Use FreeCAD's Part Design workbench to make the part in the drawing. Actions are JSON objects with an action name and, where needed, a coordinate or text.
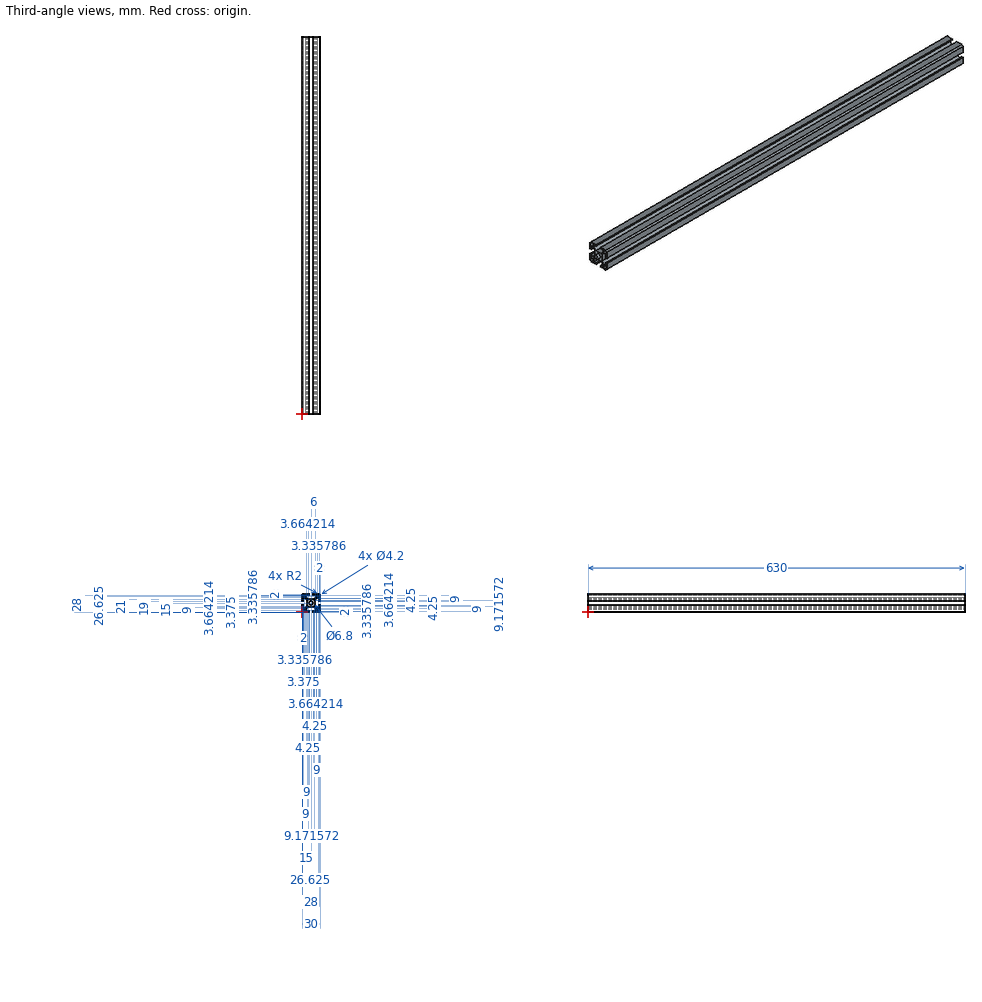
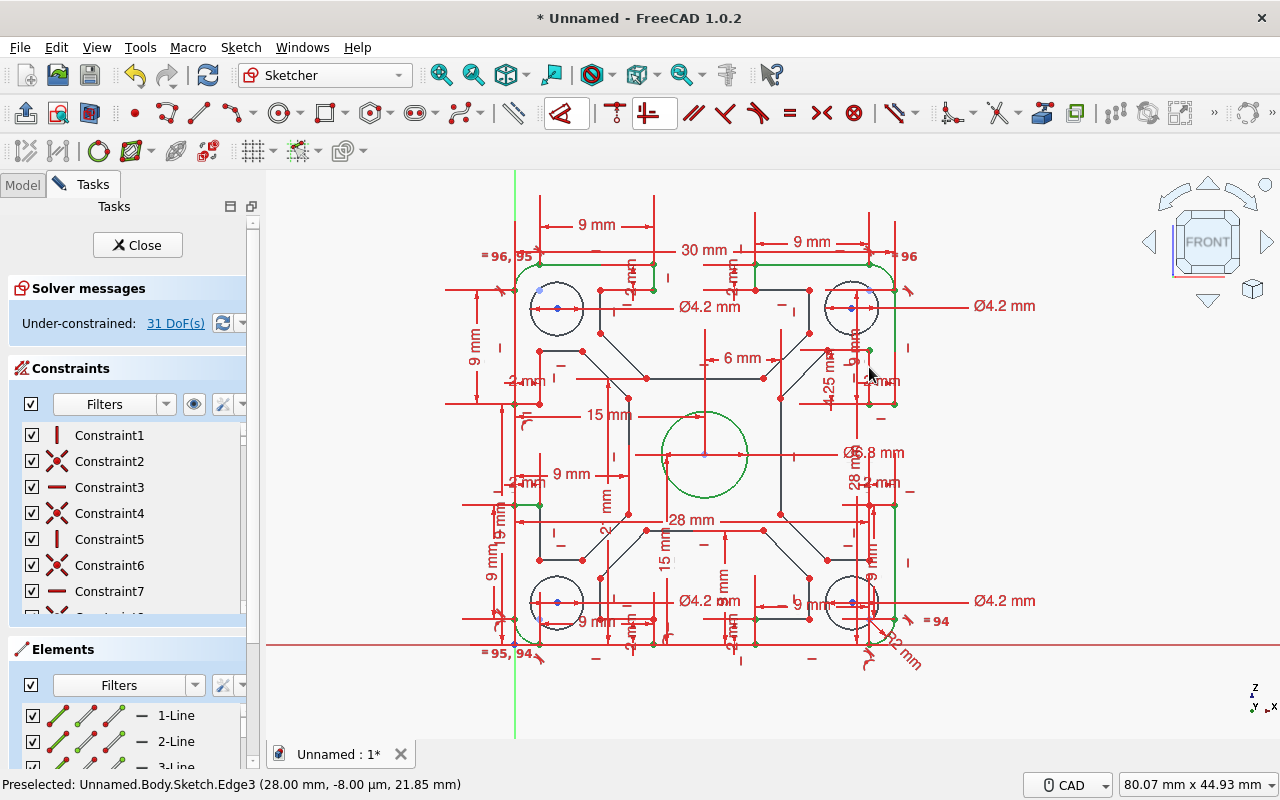
{"action": "left_click", "coordinate": [869, 522]}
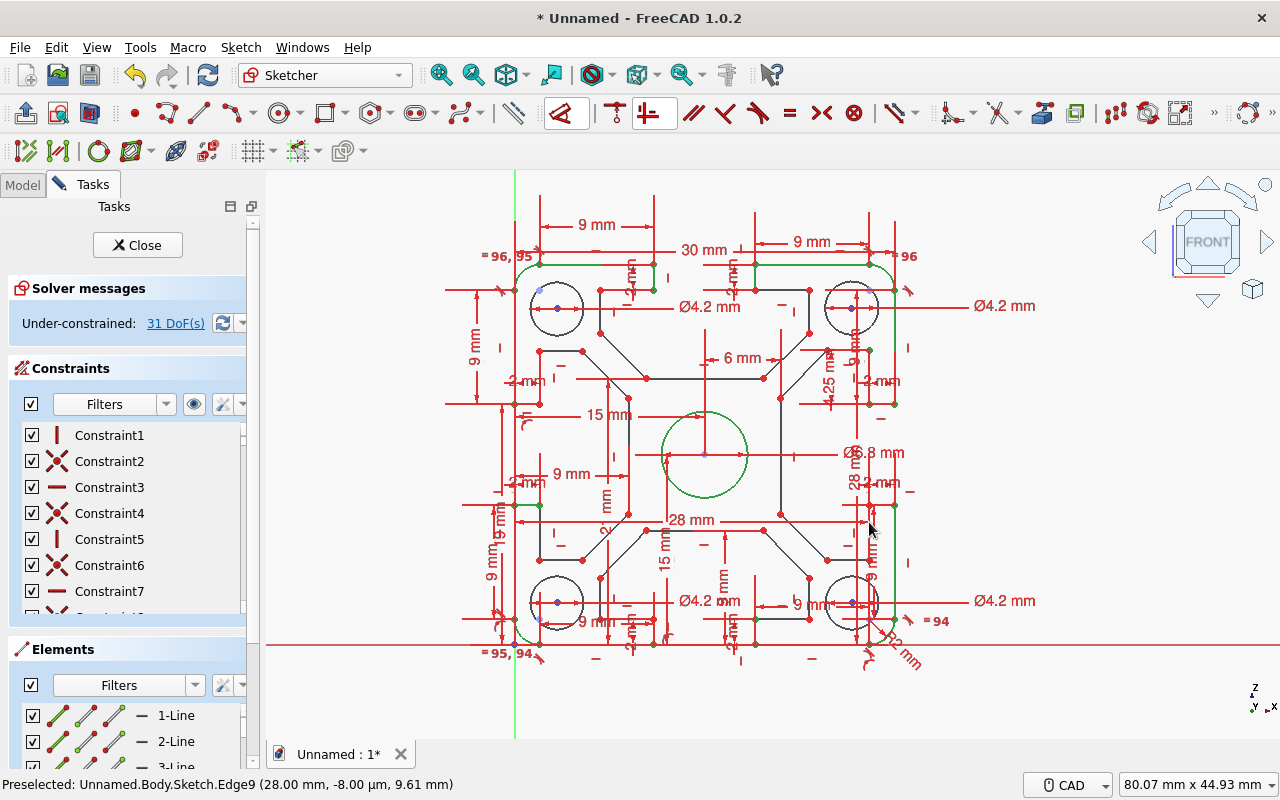
{"action": "key", "text": "i"}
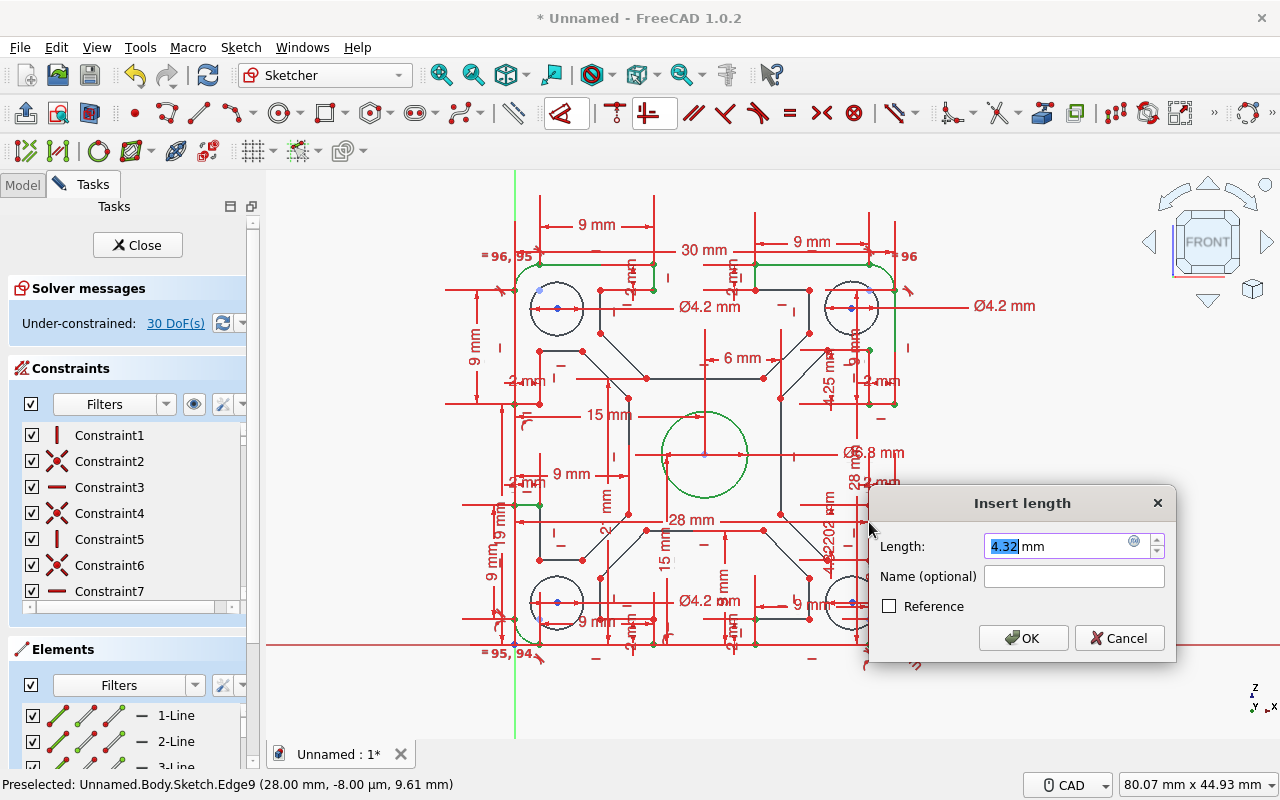
{"action": "type", "text": "4.25"}
{"action": "key", "text": "Return"}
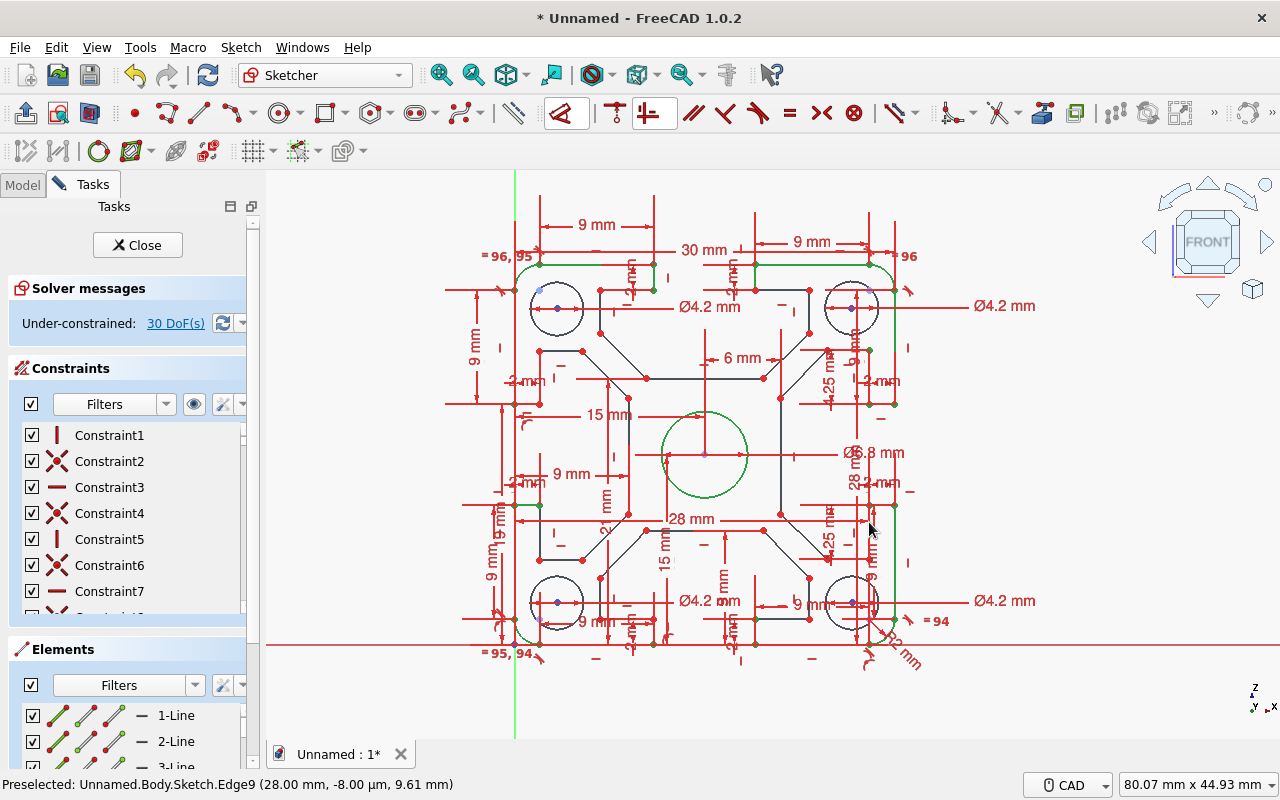
{"action": "left_click", "coordinate": [771, 619]}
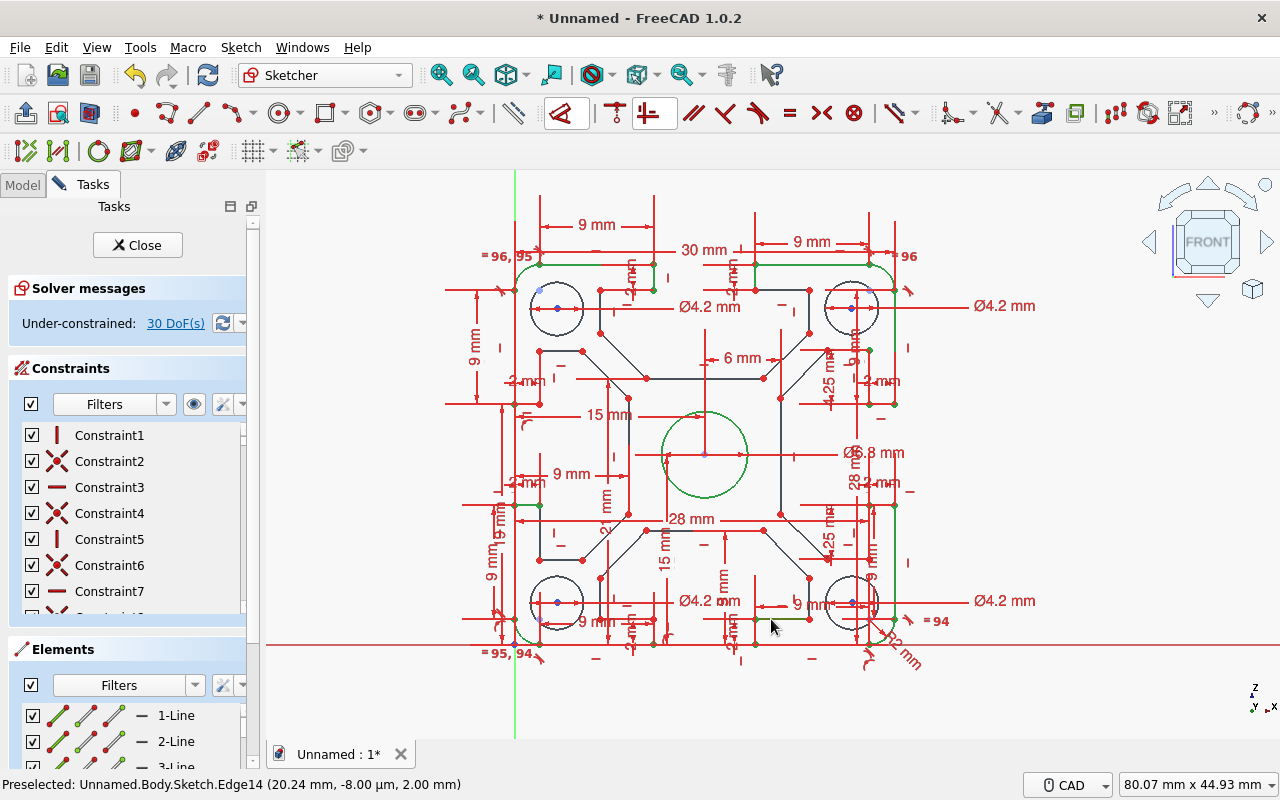
{"action": "key", "text": "l"}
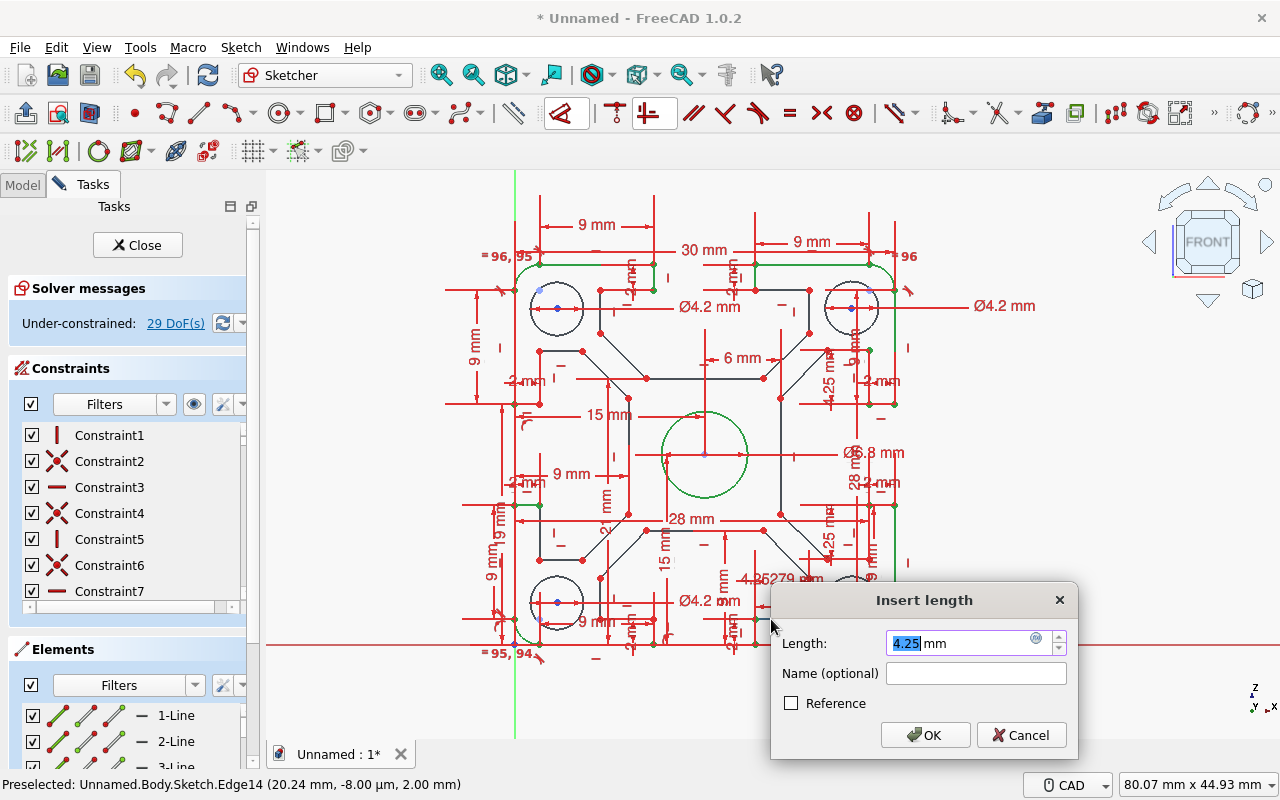
{"action": "type", "text": "4.25"}
{"action": "key", "text": "Return"}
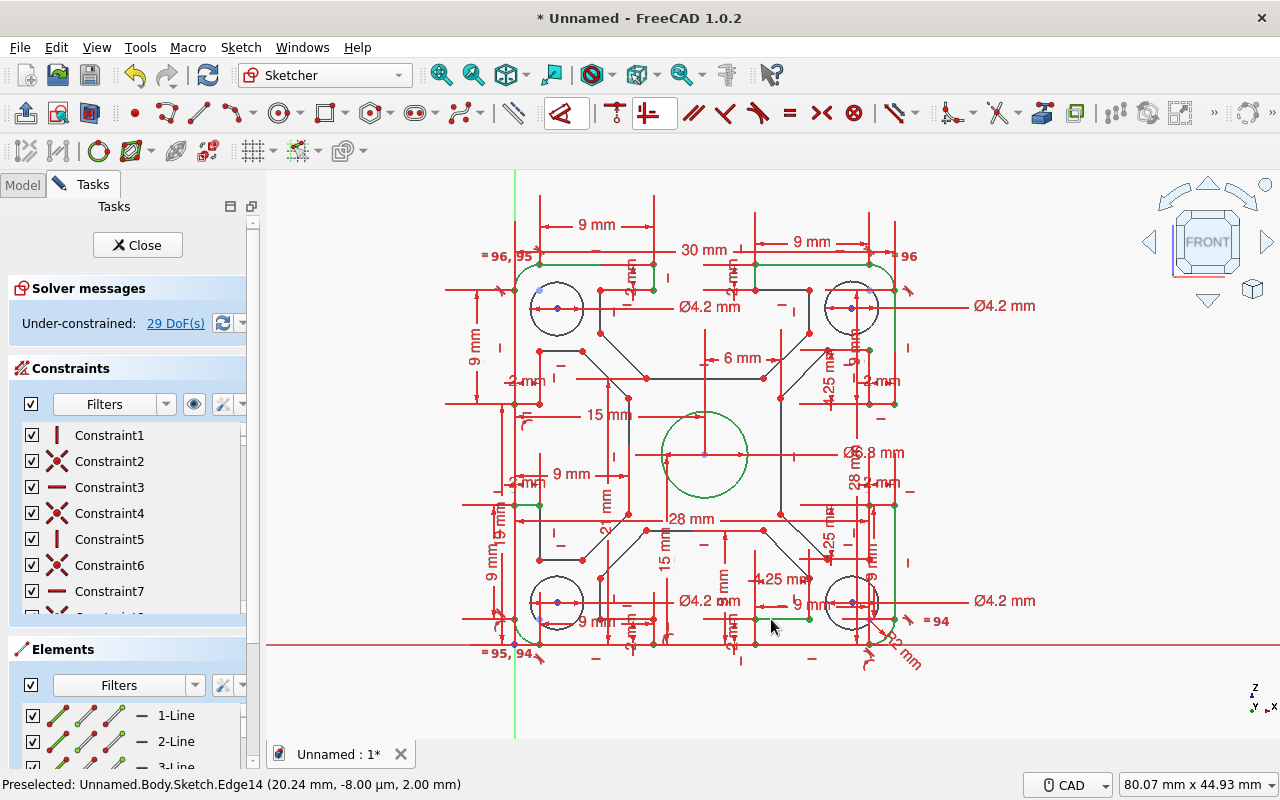
{"action": "left_click", "coordinate": [616, 619]}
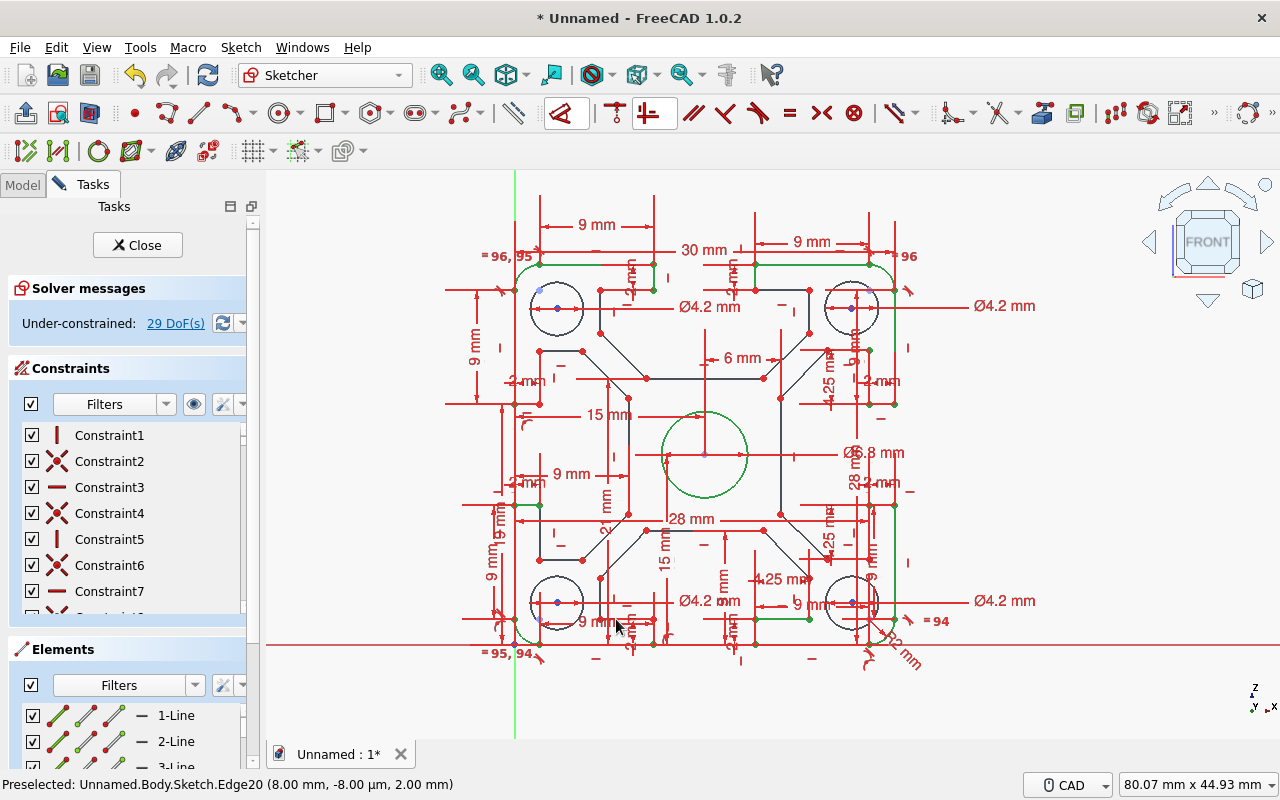
{"action": "key", "text": "l"}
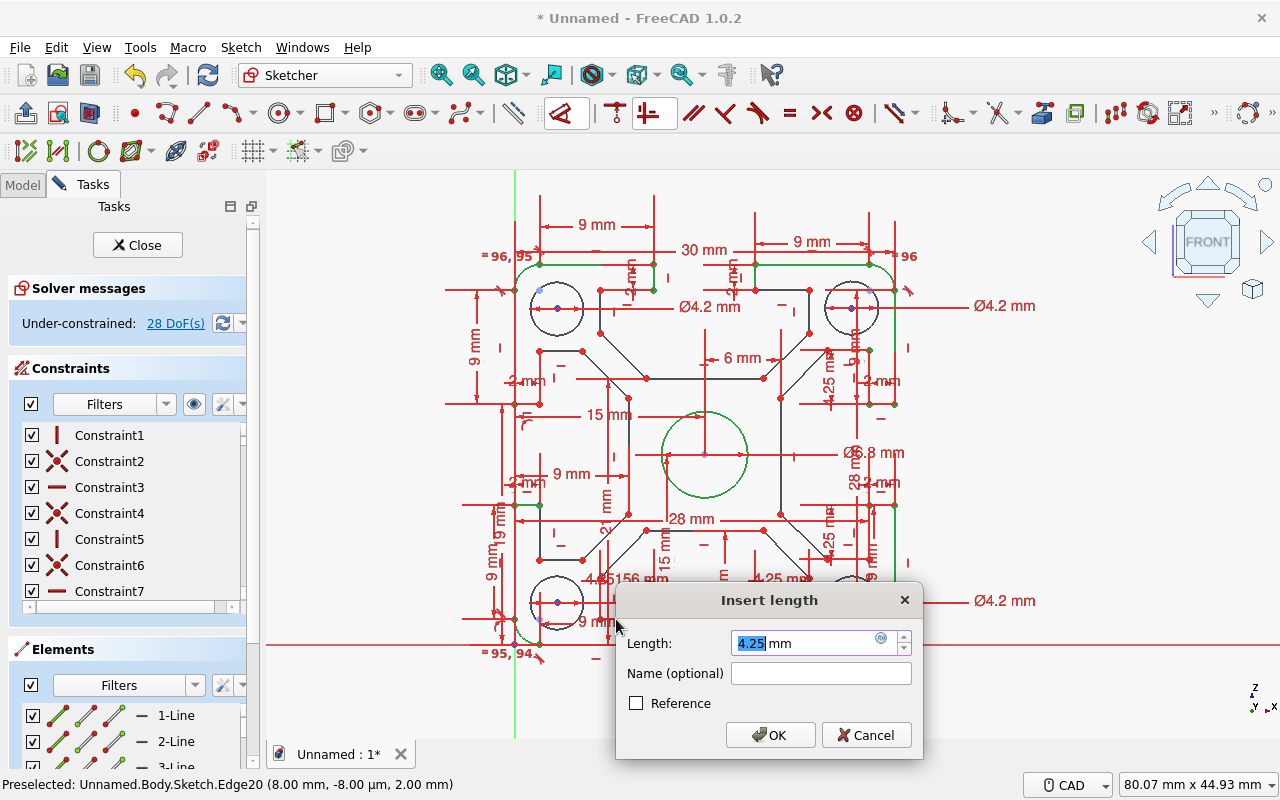
{"action": "type", "text": "4.25"}
{"action": "key", "text": "Return"}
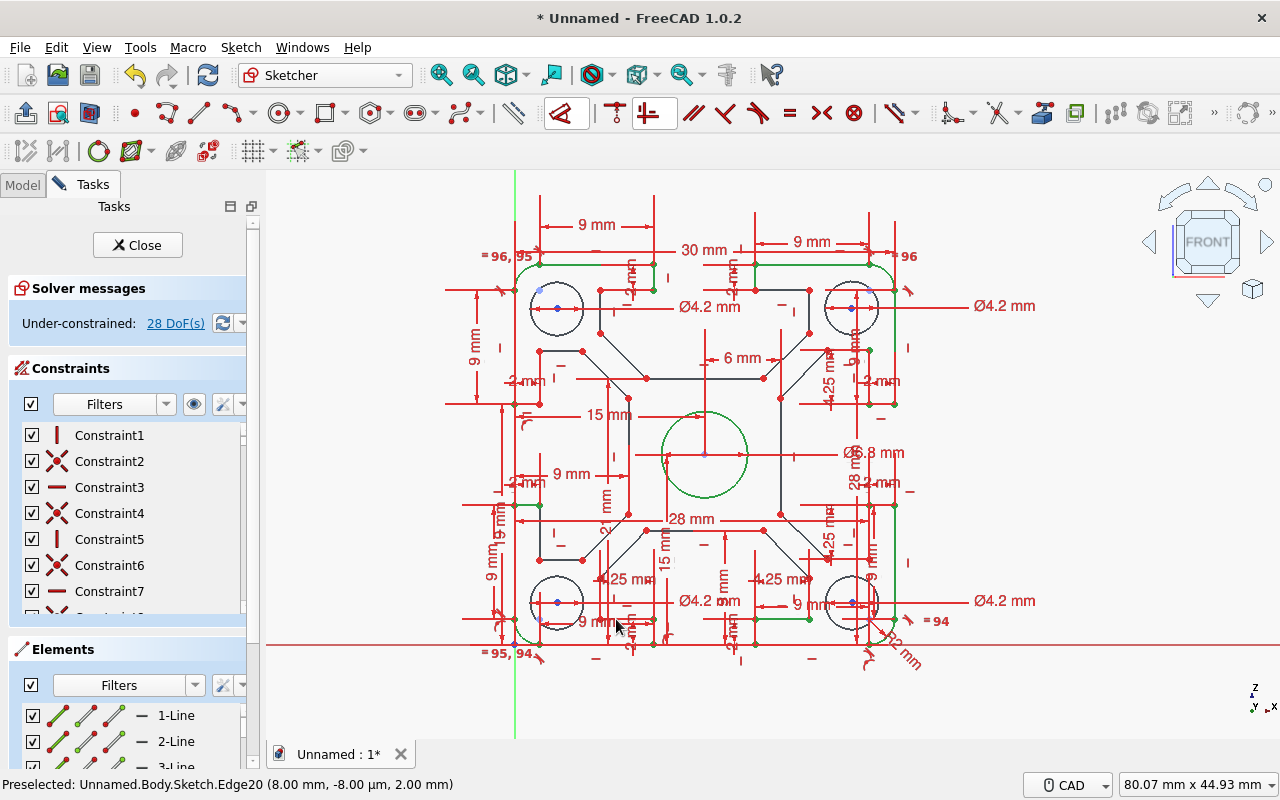
{"action": "left_click", "coordinate": [540, 522]}